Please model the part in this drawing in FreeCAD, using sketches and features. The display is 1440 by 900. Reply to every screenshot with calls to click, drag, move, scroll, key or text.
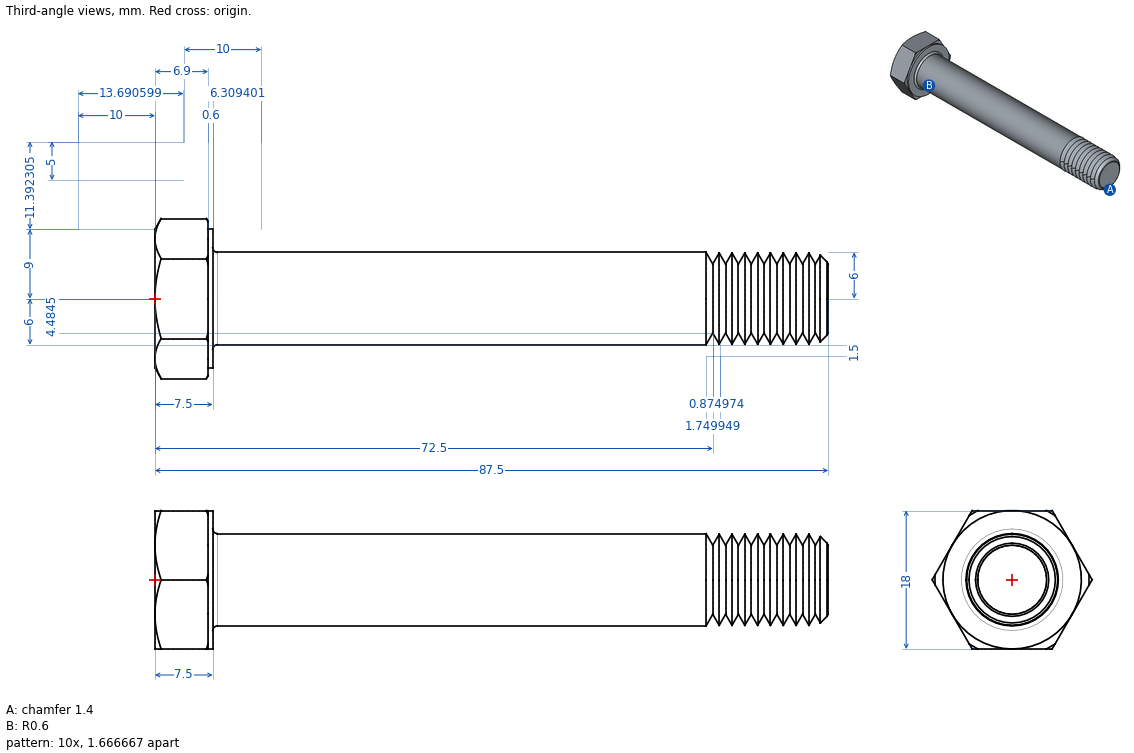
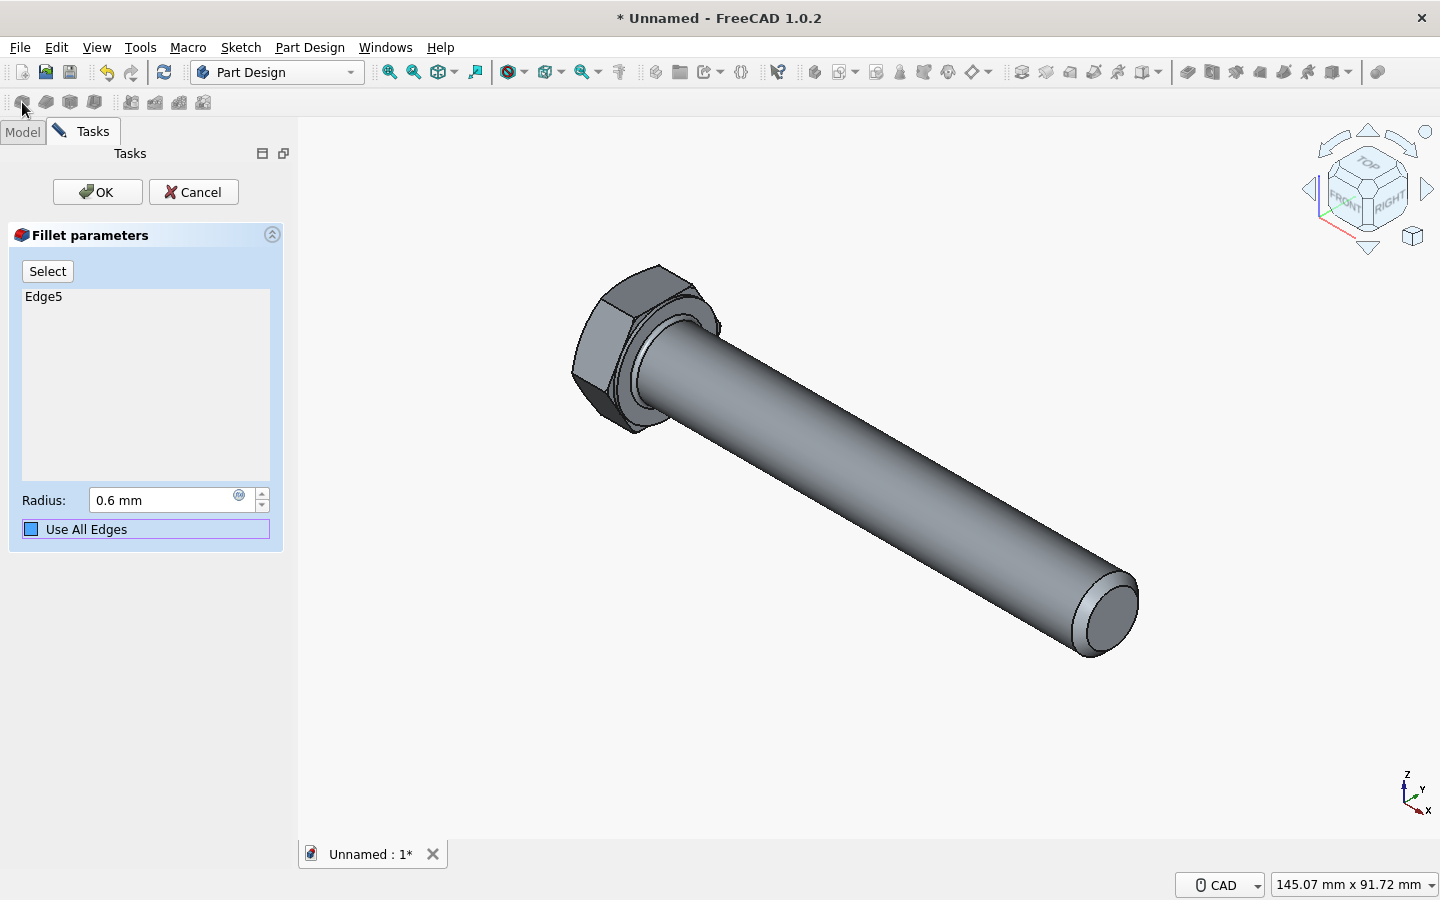
click(98, 192)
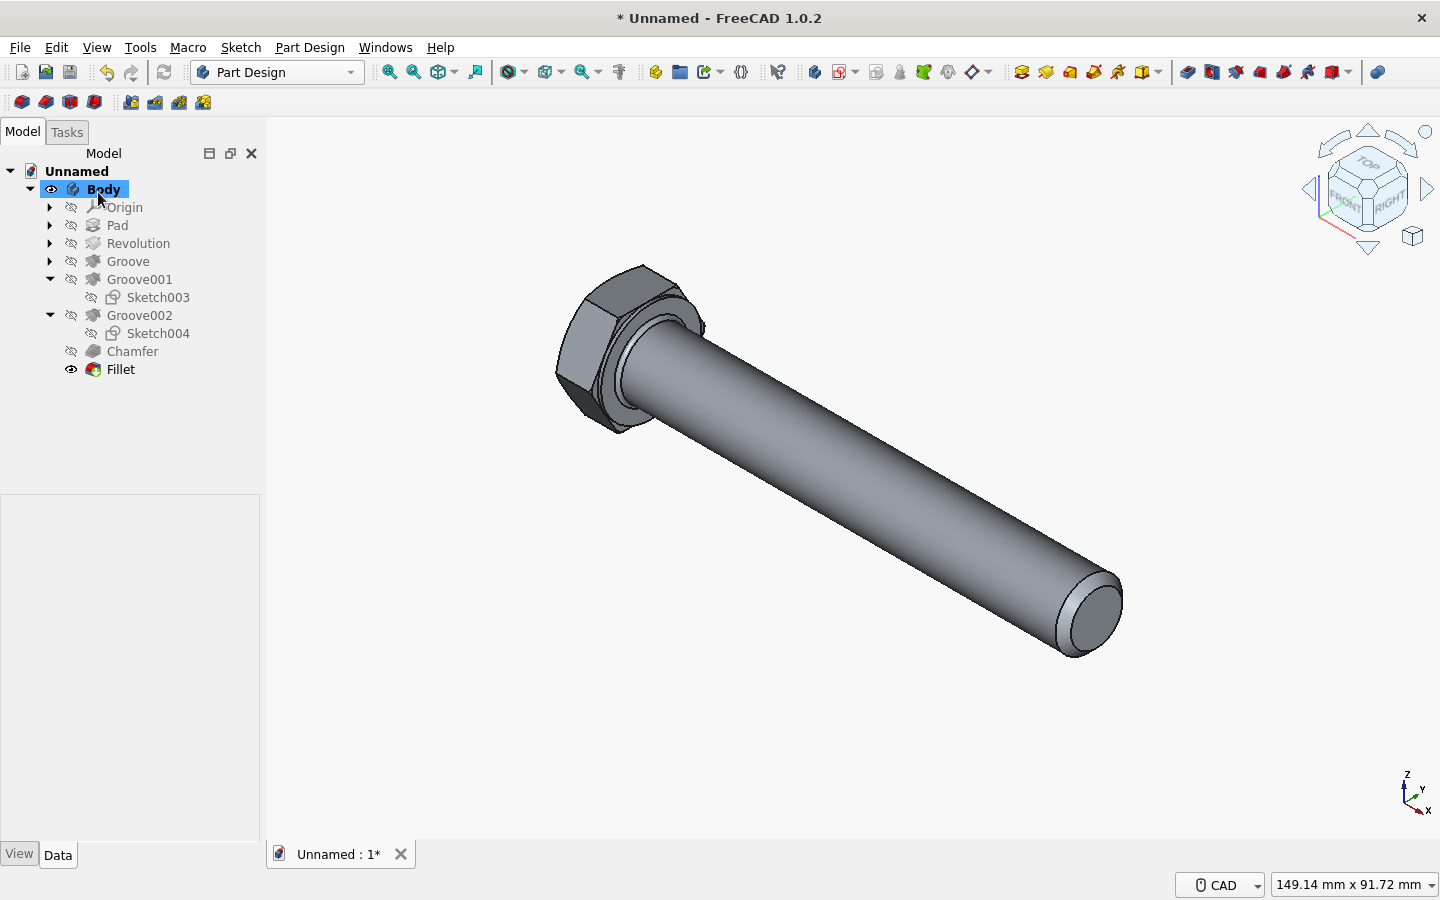
click(840, 72)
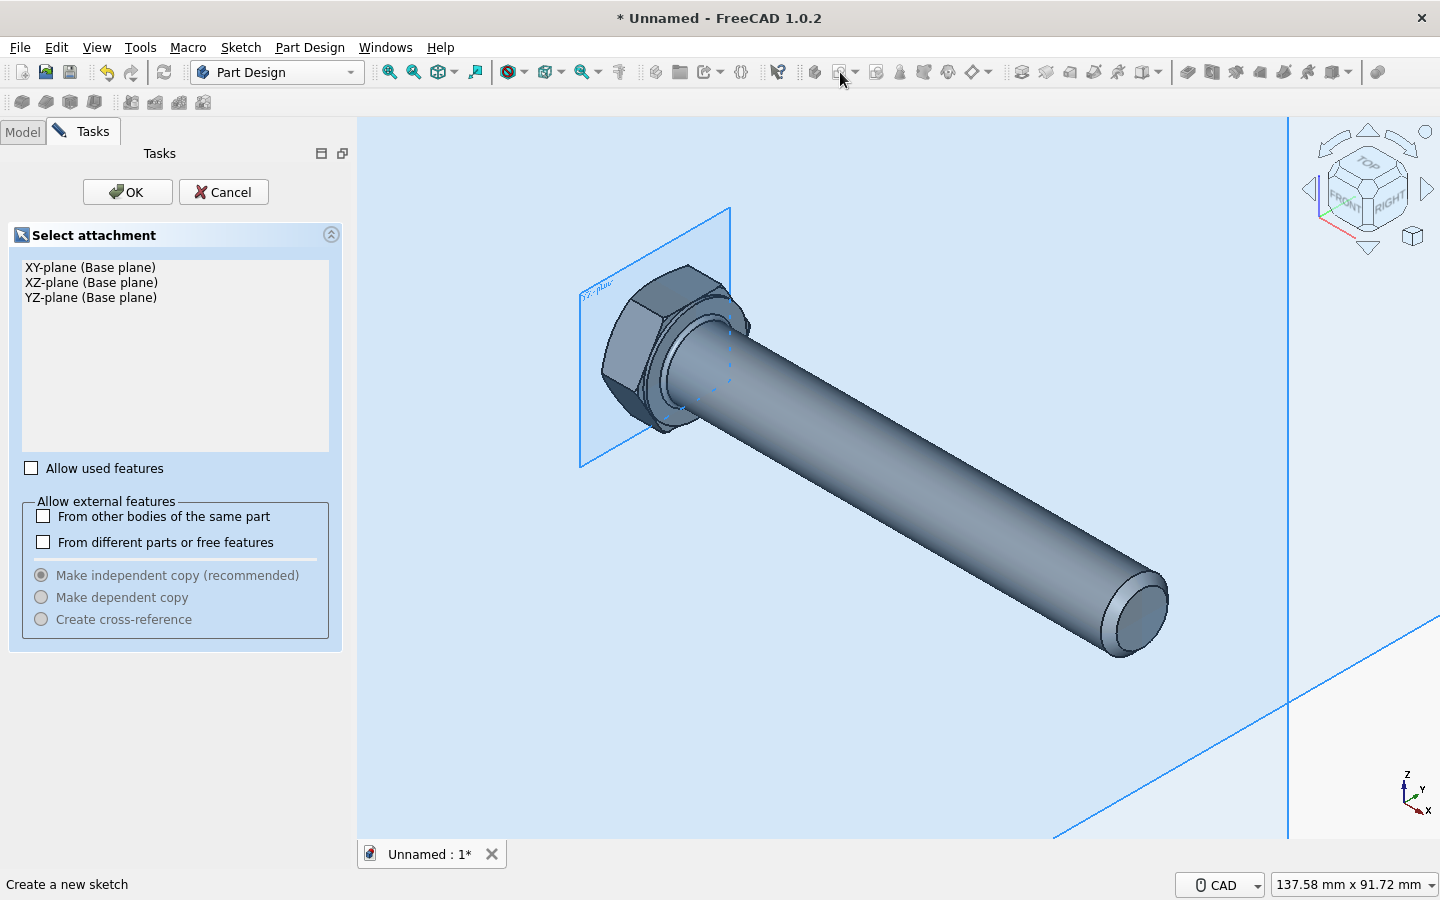
click(82, 268)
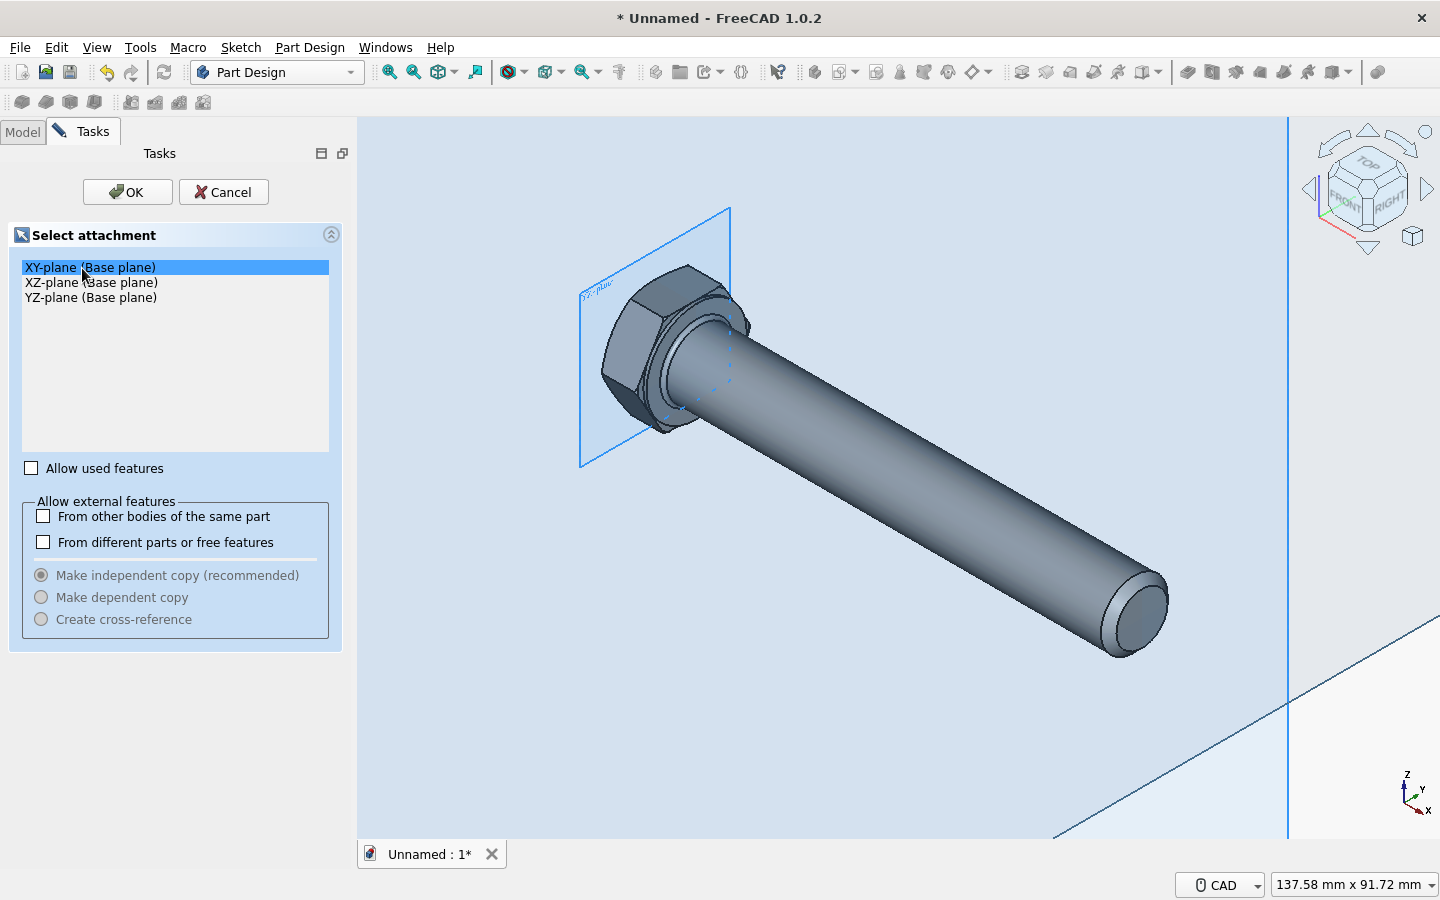
click(128, 192)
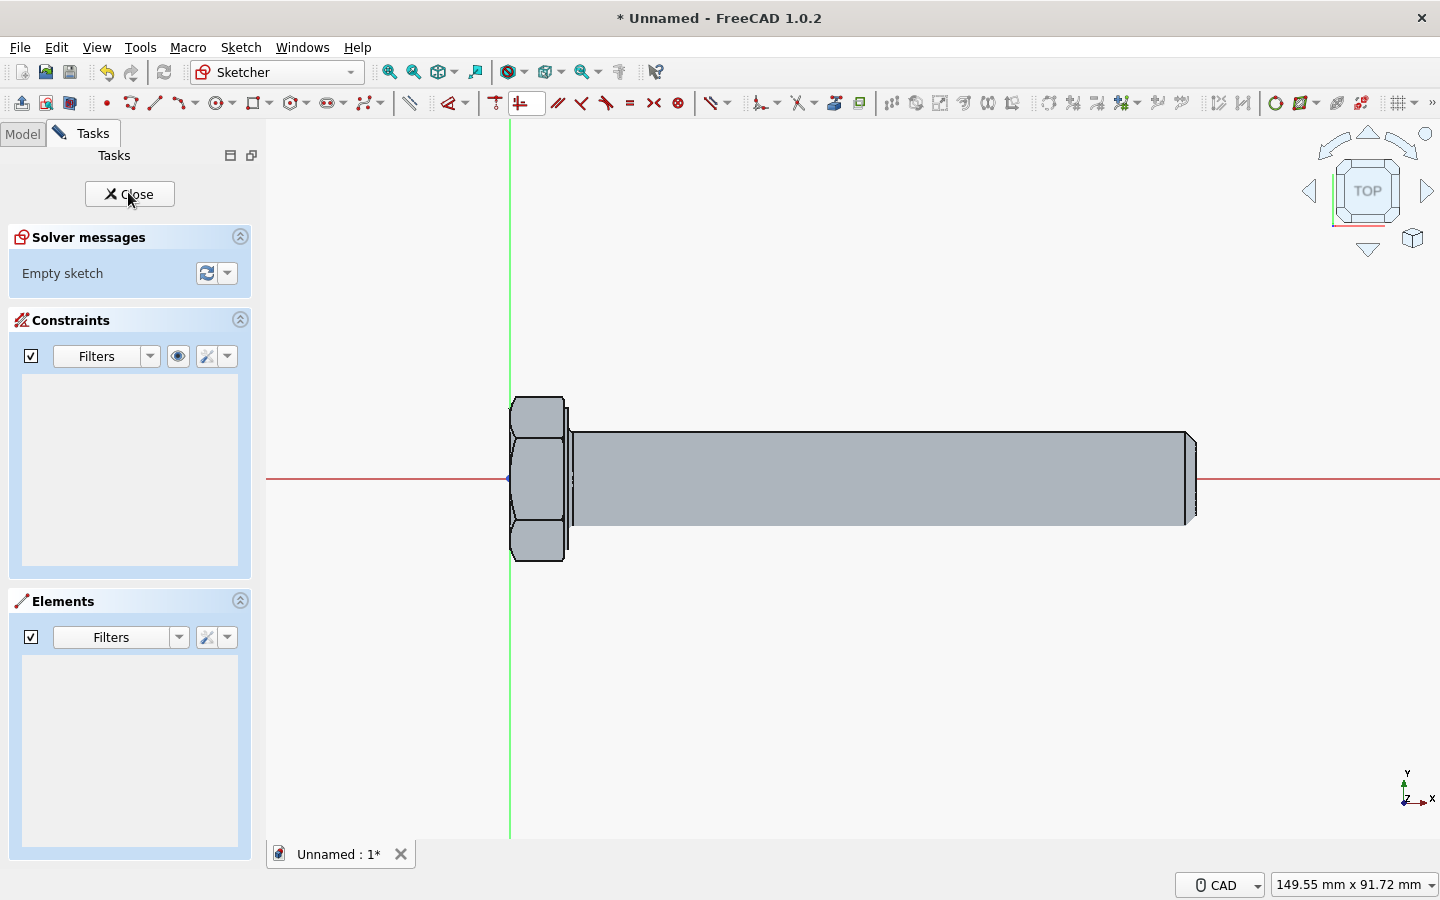
click(70, 104)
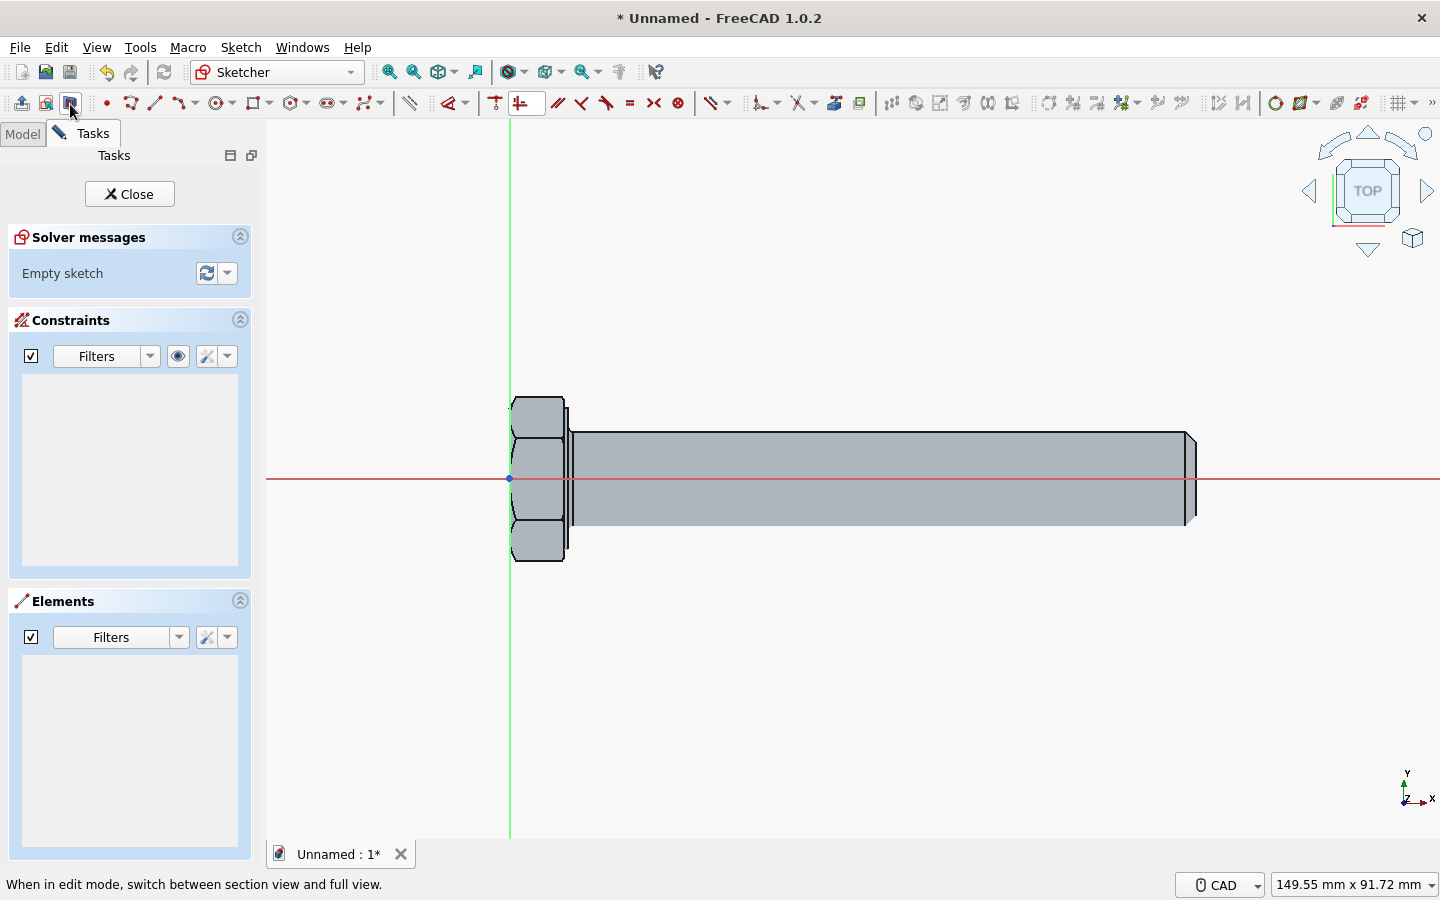
scroll(1094, 529, up, 15)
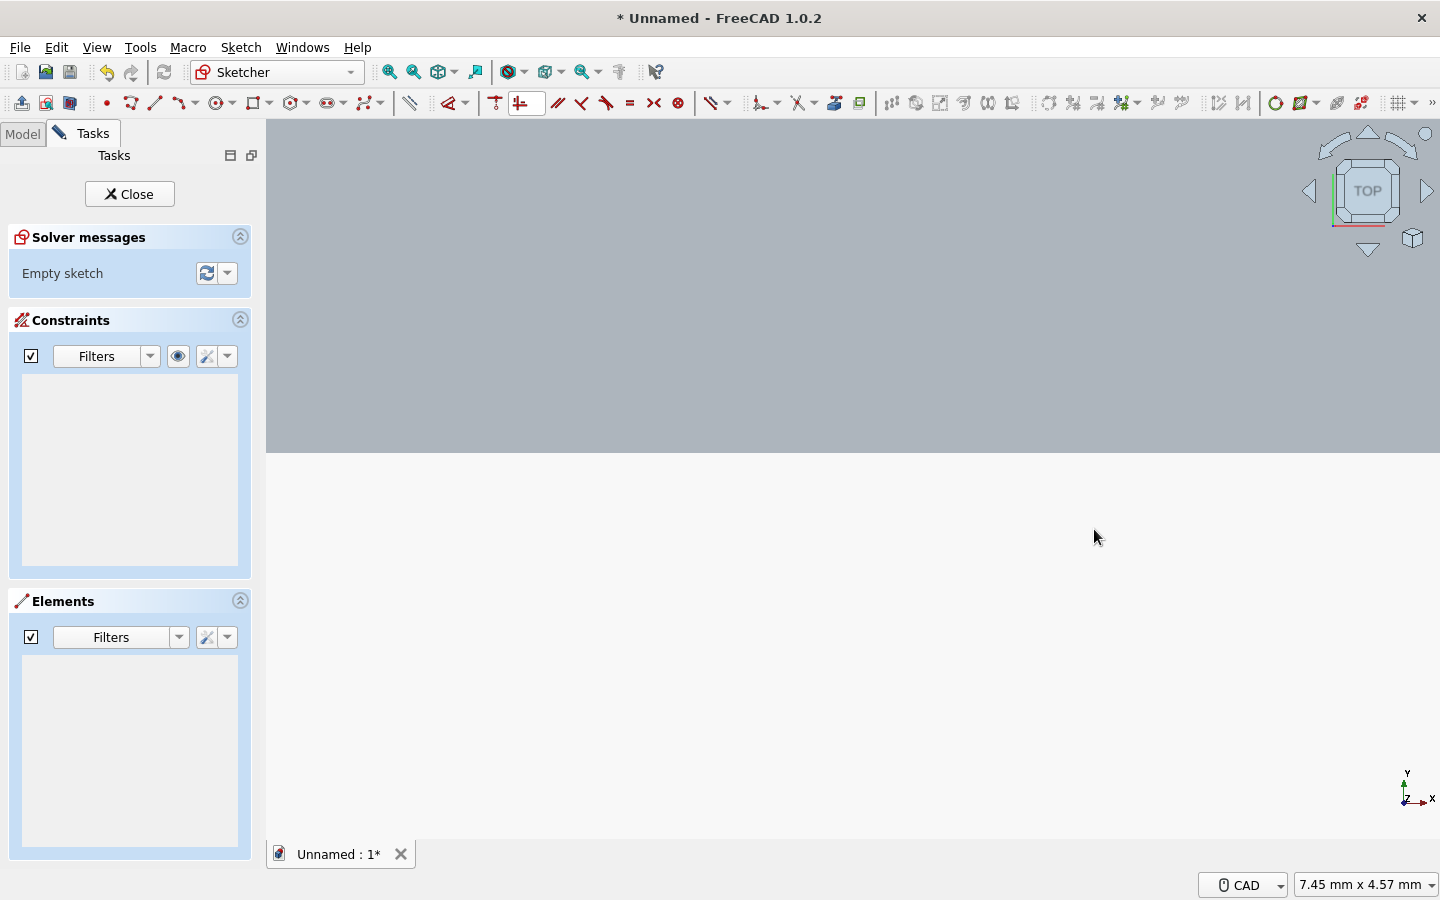
click(132, 104)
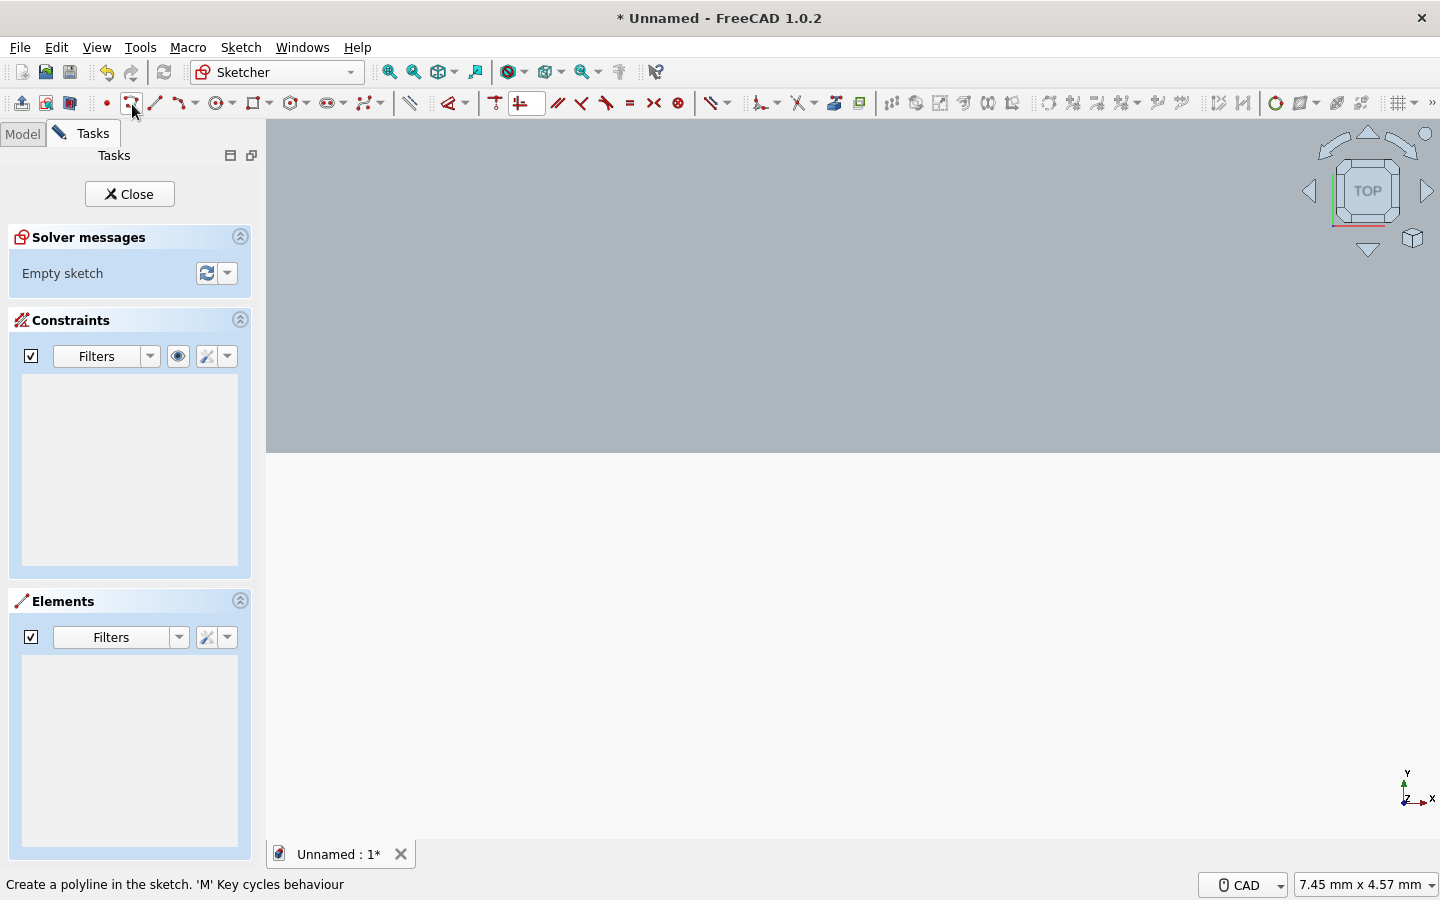
click(635, 460)
click(635, 696)
click(911, 696)
click(911, 460)
click(773, 221)
click(635, 461)
key(Escape)
key(Escape)